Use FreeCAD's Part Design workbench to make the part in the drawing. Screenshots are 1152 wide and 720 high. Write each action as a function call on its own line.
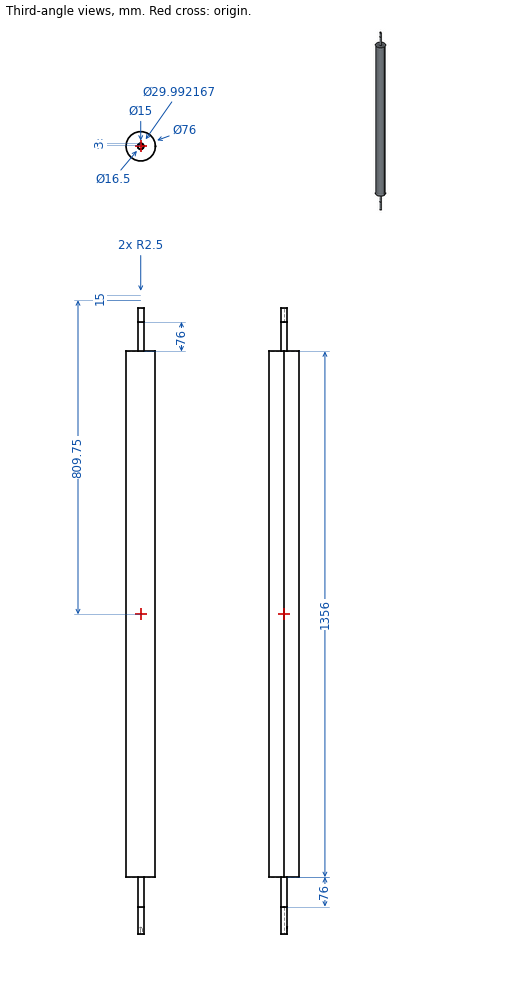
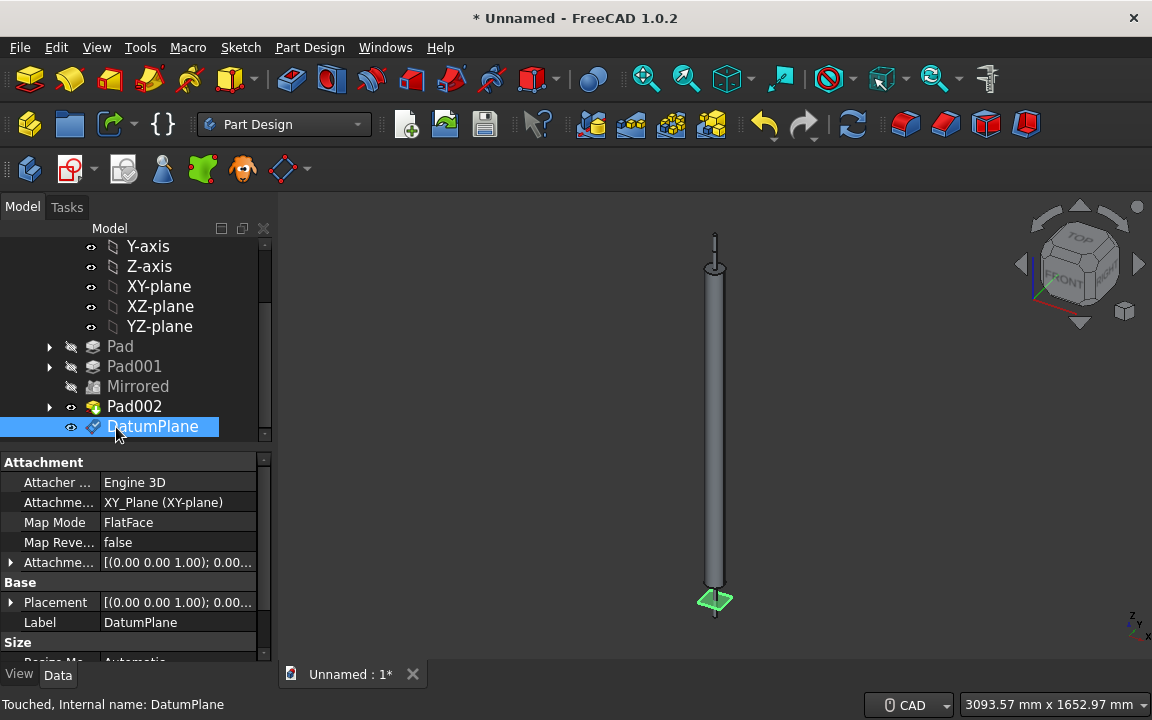
click(70, 170)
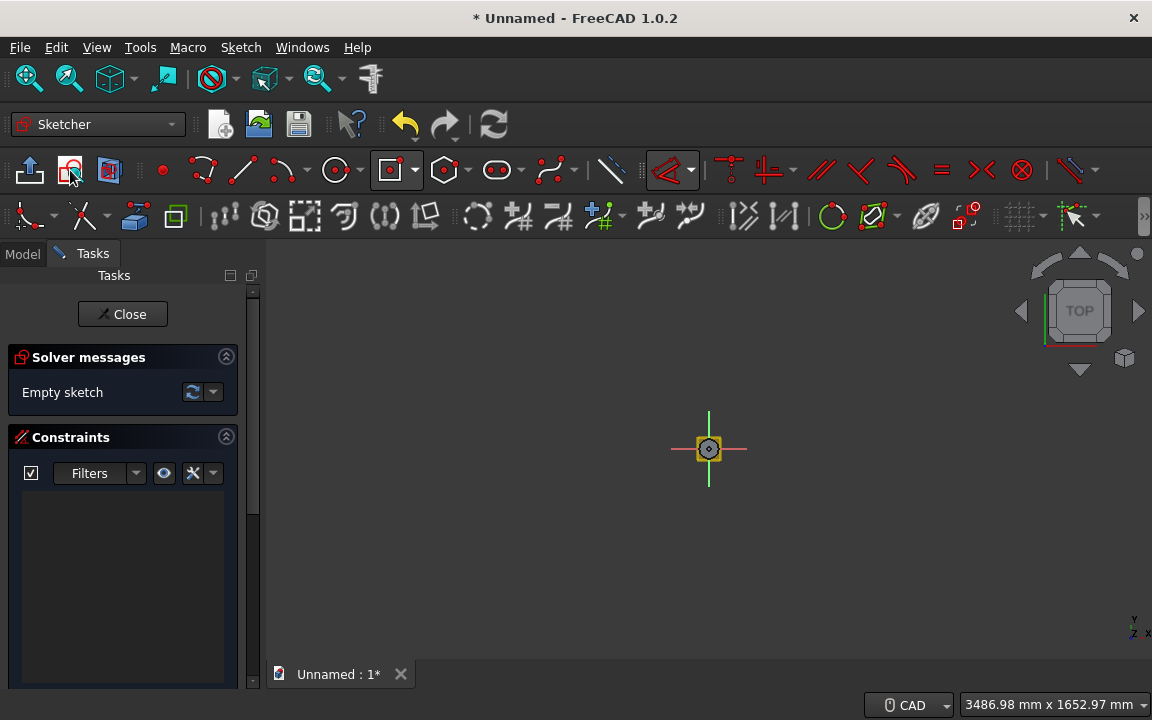
click(110, 170)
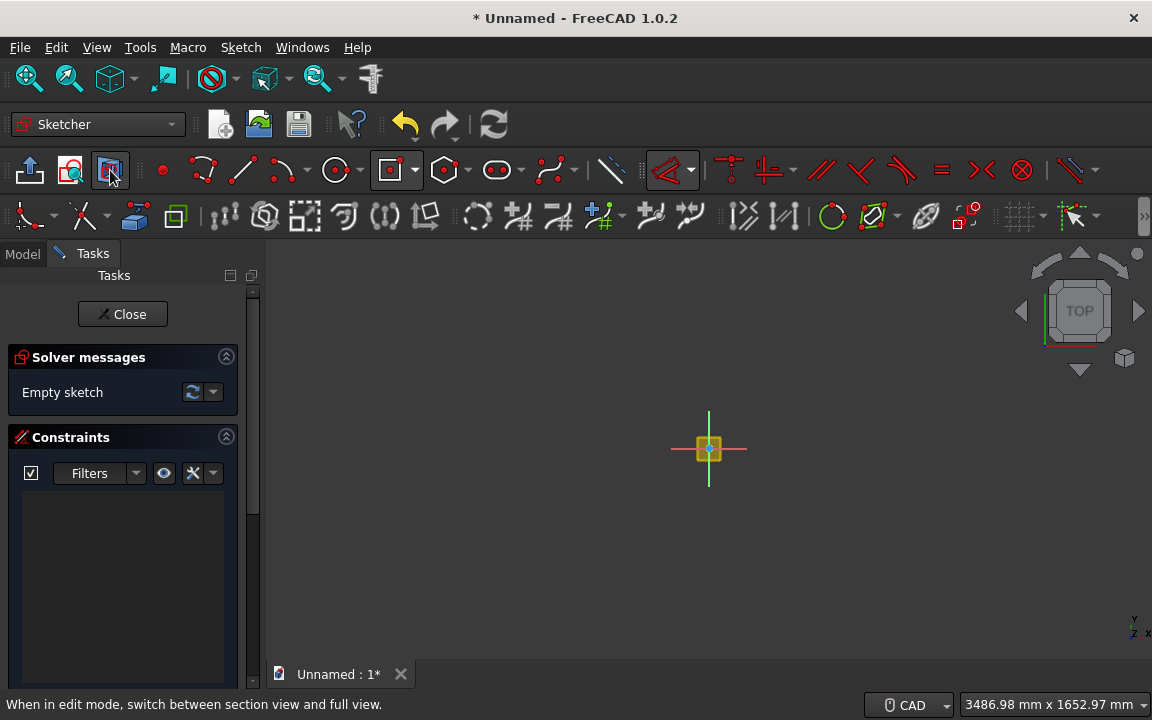
scroll(713, 449, up, 15)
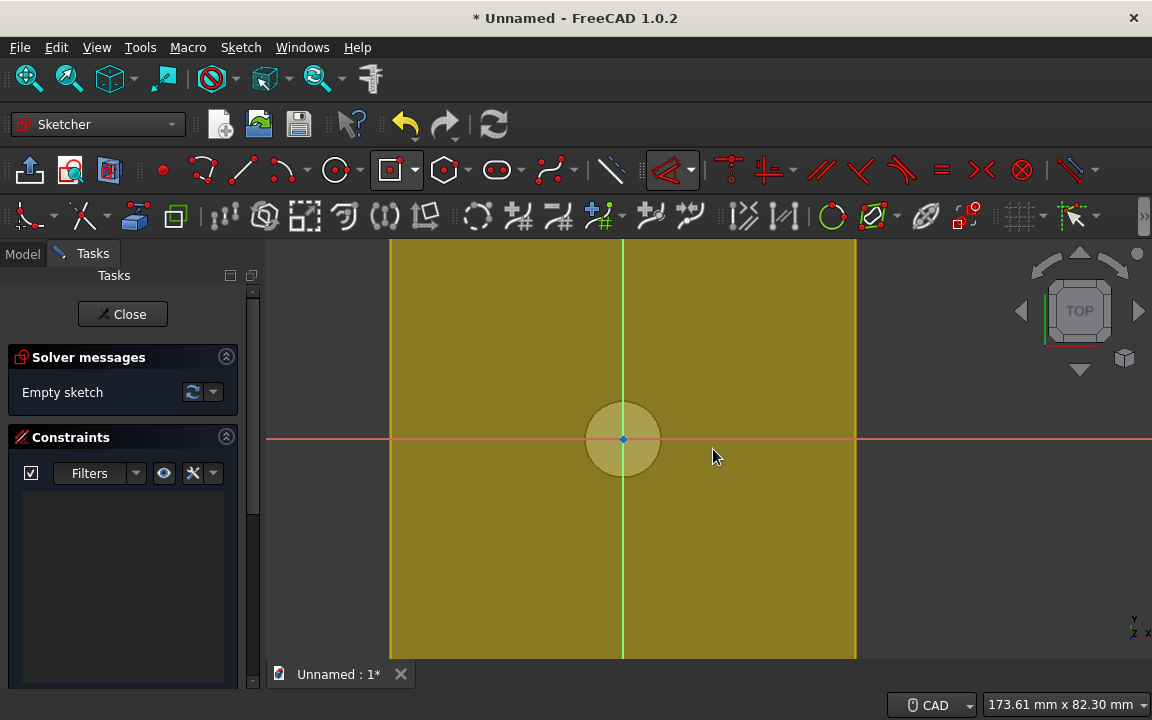
scroll(615, 435, up, 6)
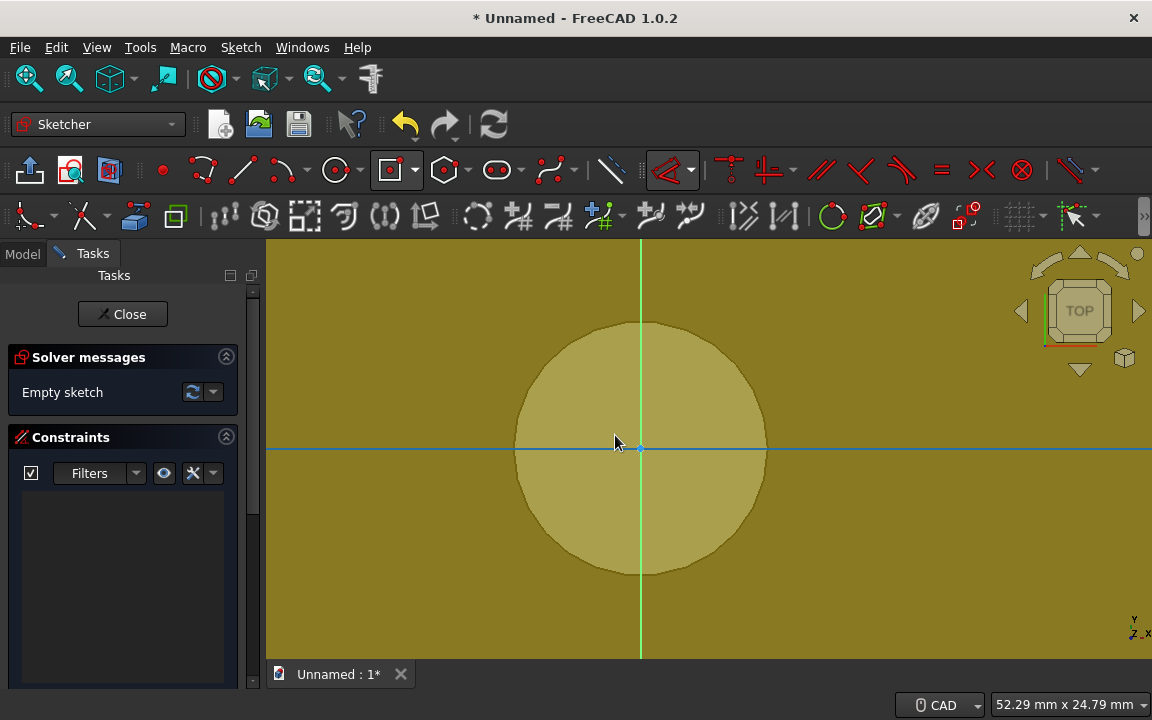
click(336, 170)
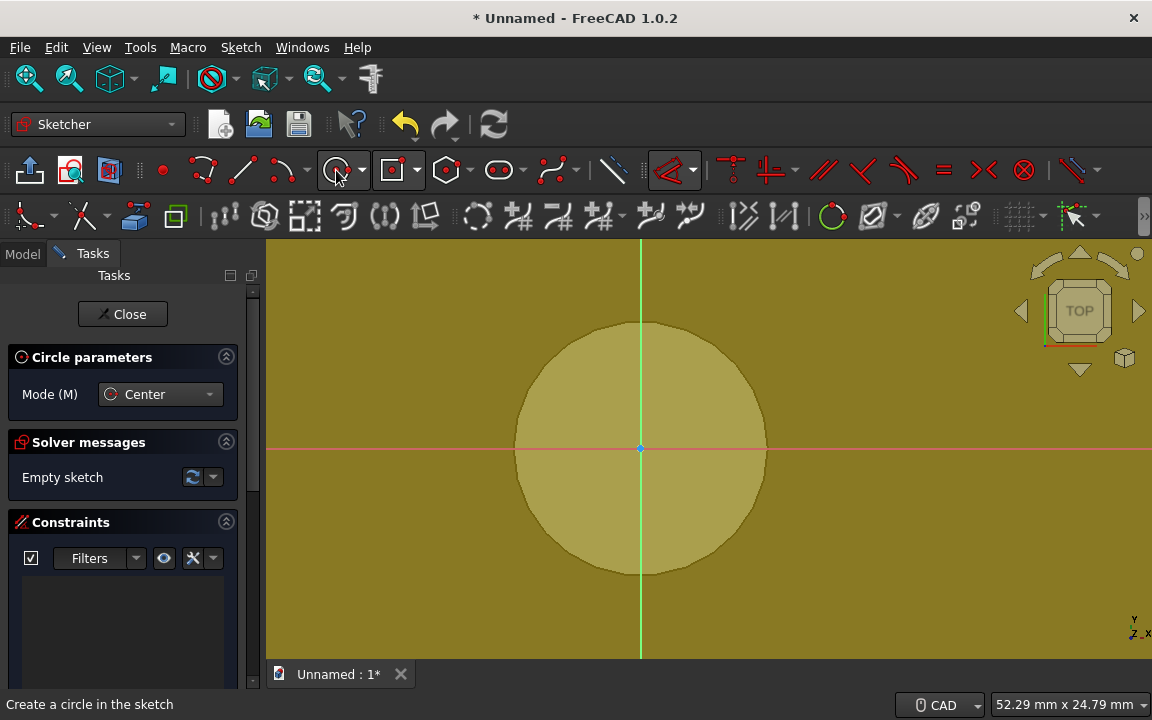
click(641, 449)
click(740, 350)
key(Escape)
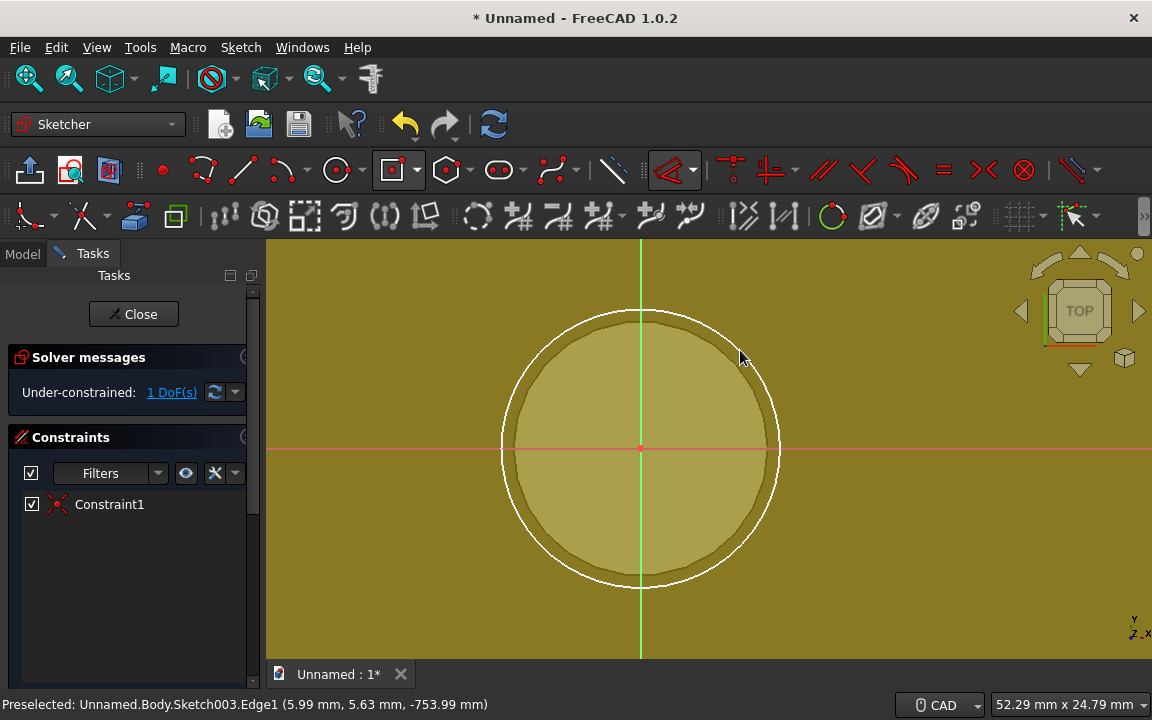
click(739, 350)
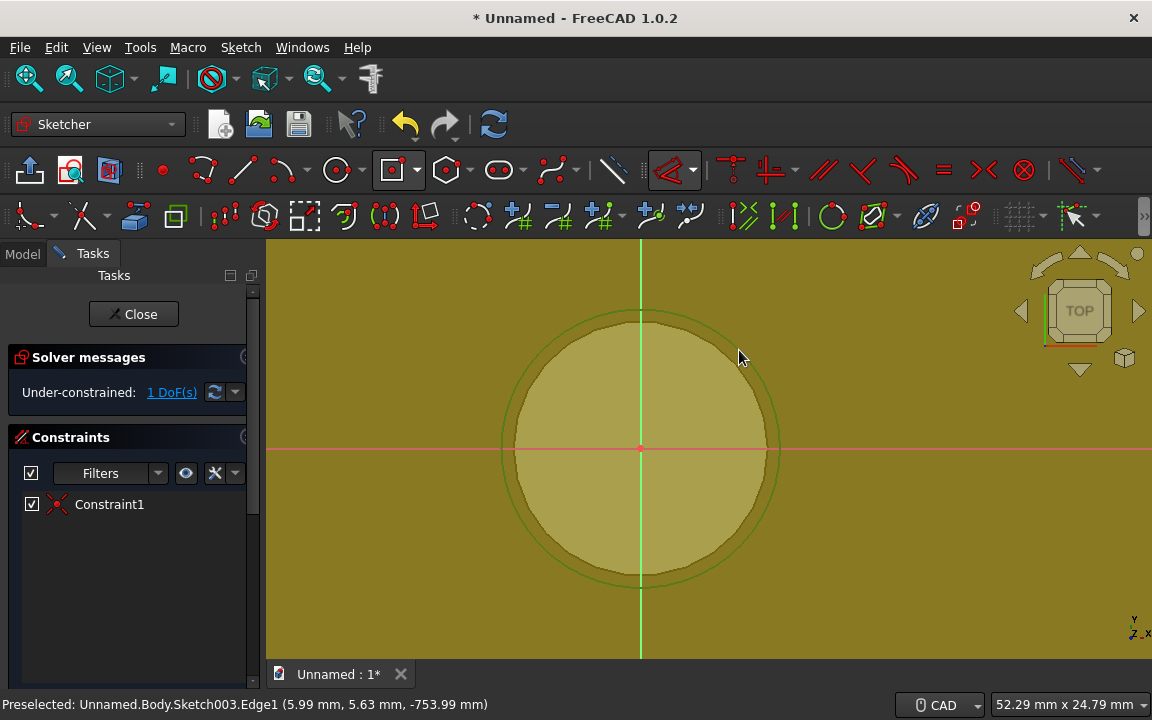
click(696, 170)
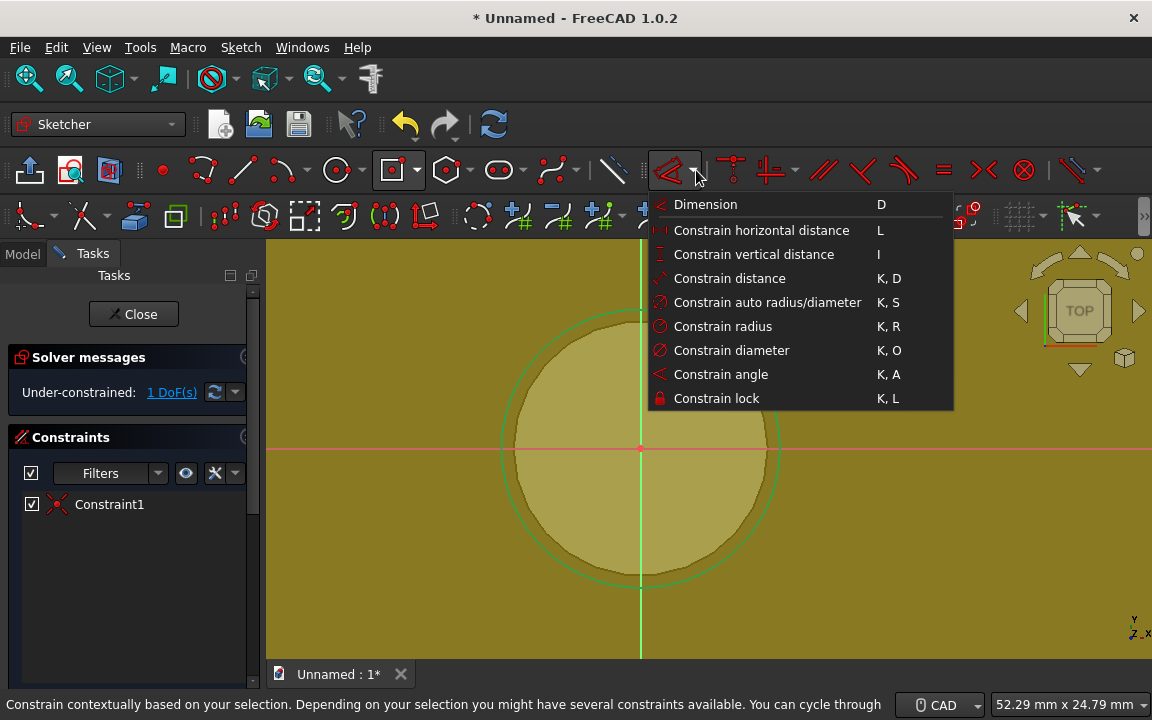
click(801, 350)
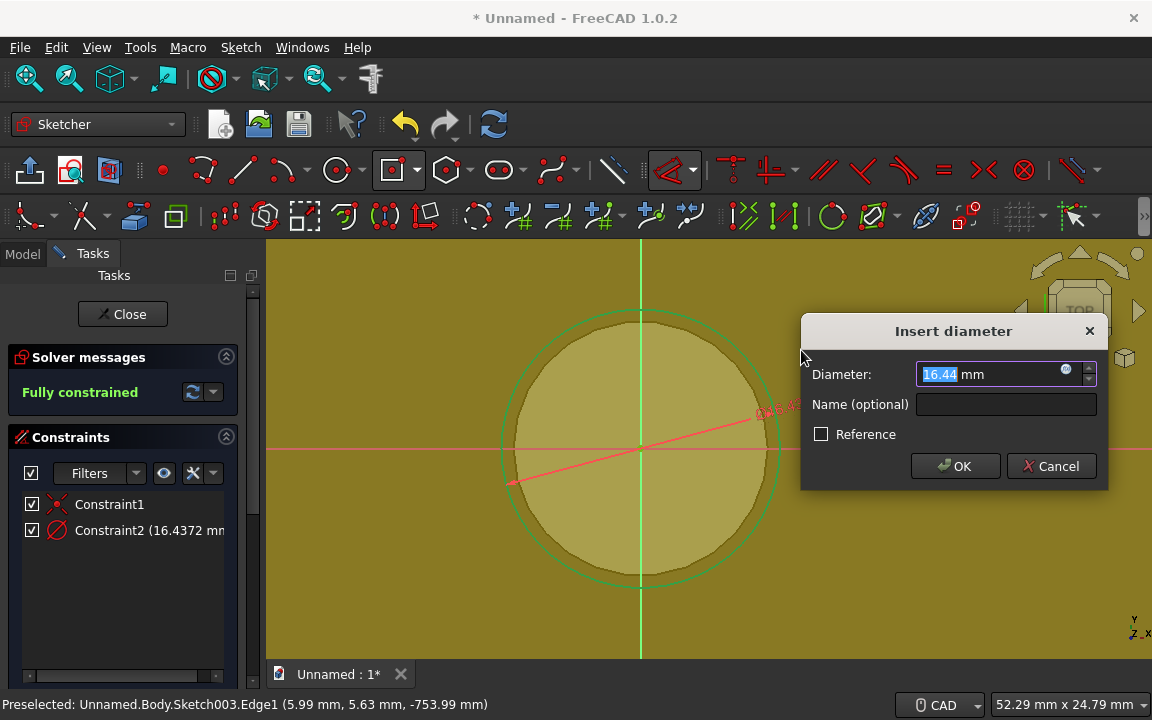
text(16.5)
key(Return)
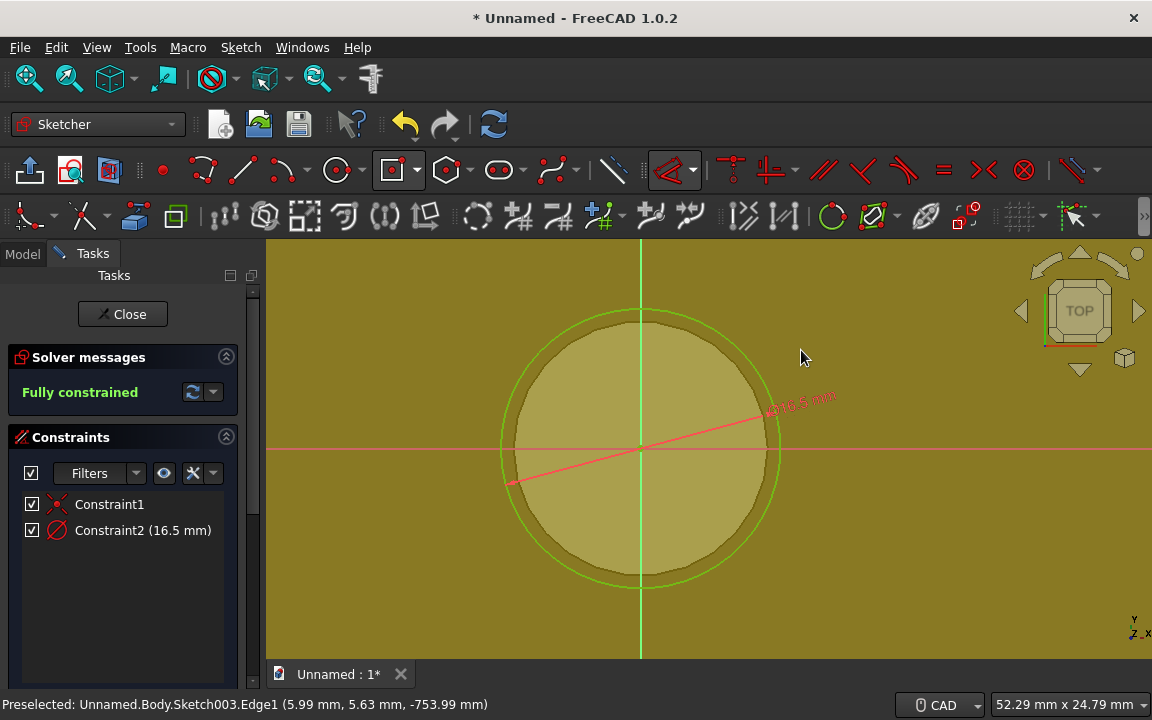
click(123, 314)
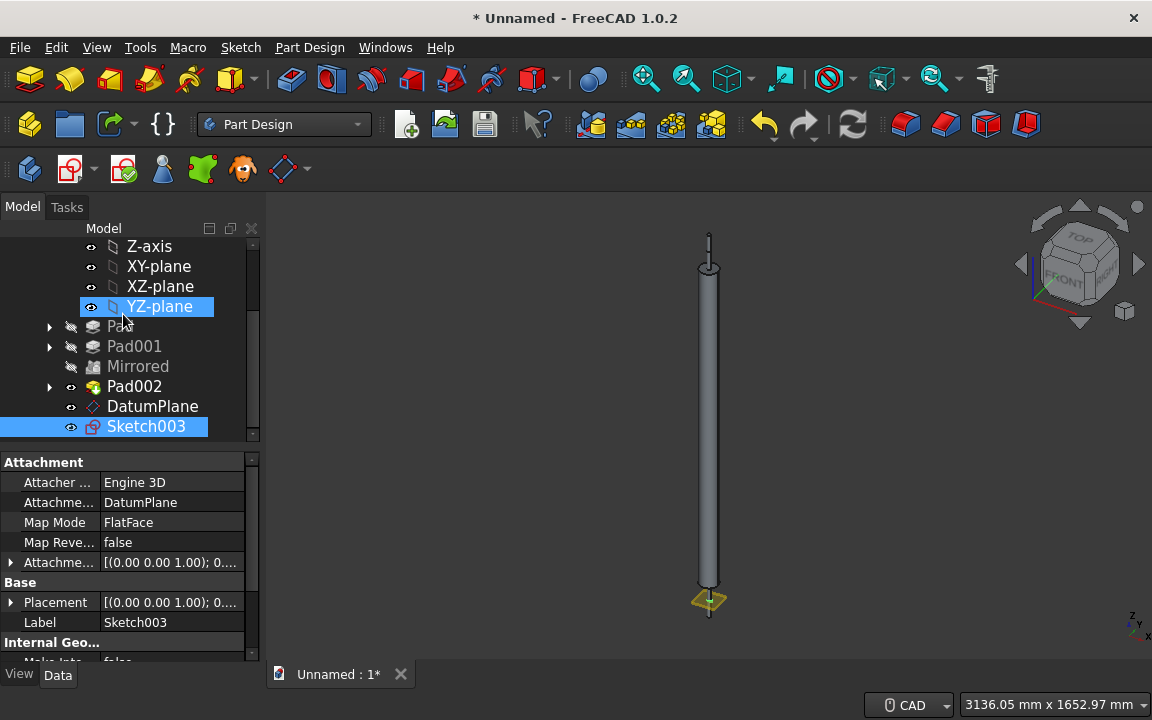
click(30, 80)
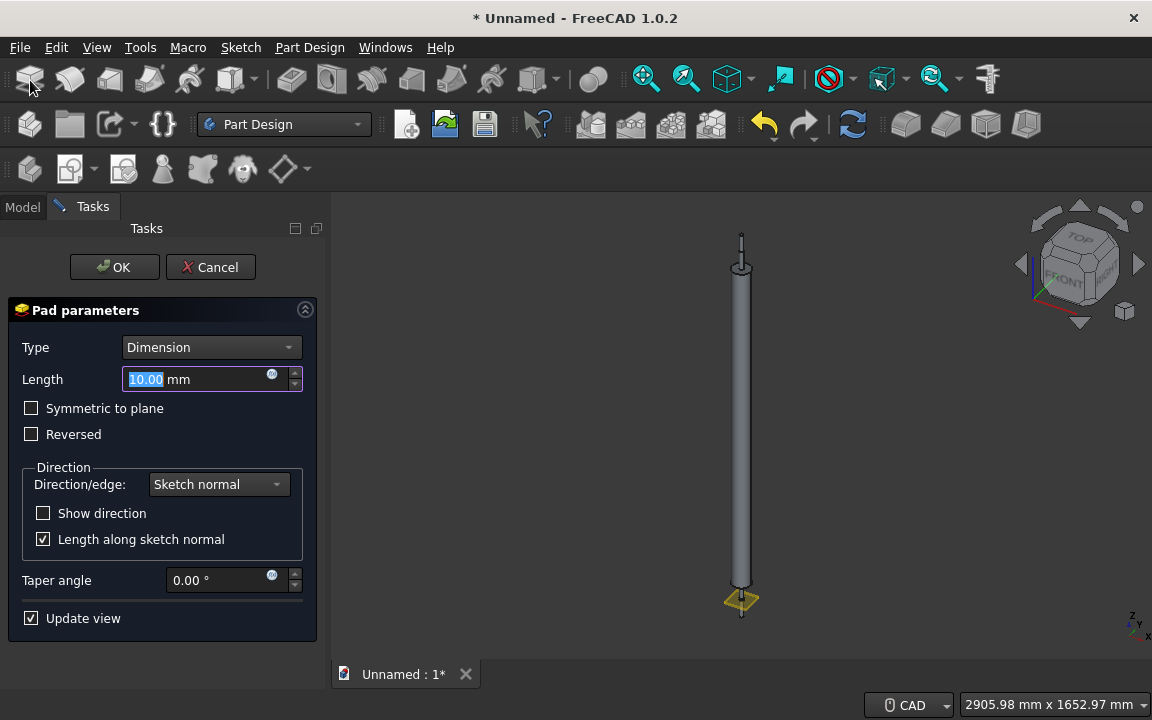
text(76)
key(Tab)